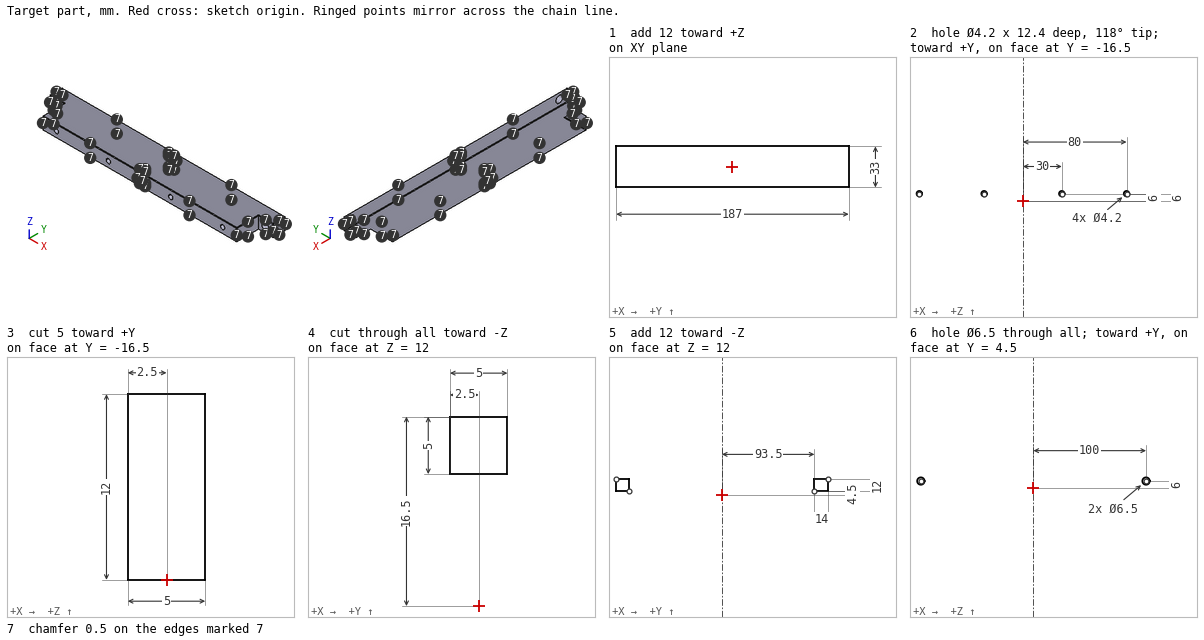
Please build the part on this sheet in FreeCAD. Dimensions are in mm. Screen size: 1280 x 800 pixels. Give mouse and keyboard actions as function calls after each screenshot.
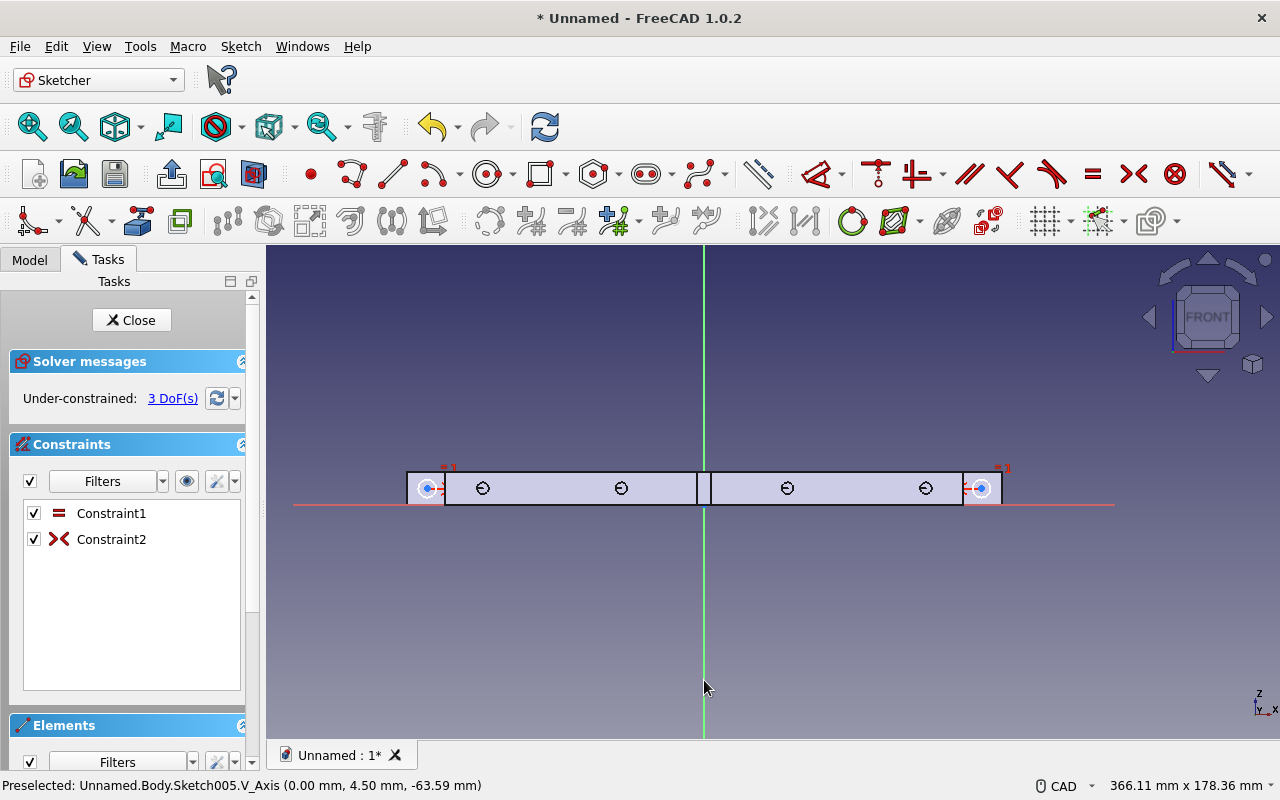
click(816, 174)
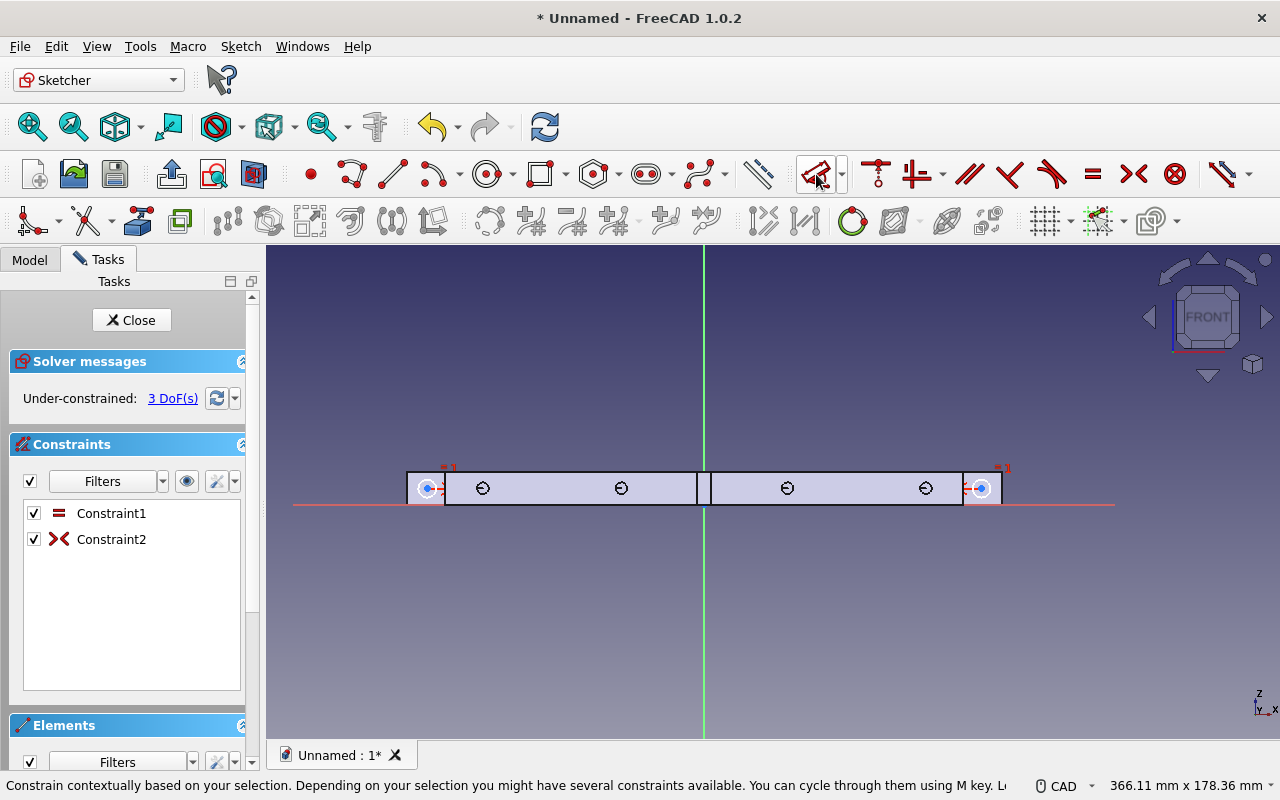
scroll(988, 495, up, 4)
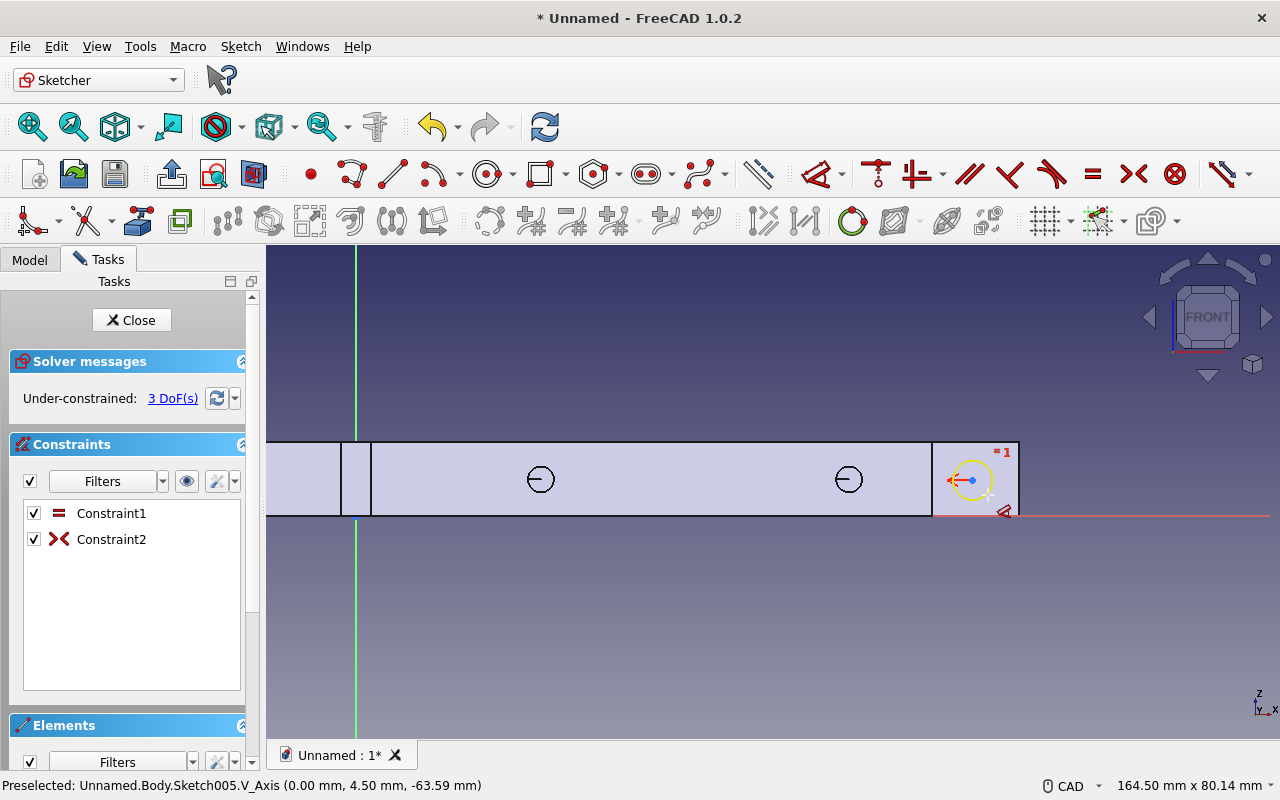
click(987, 494)
click(988, 530)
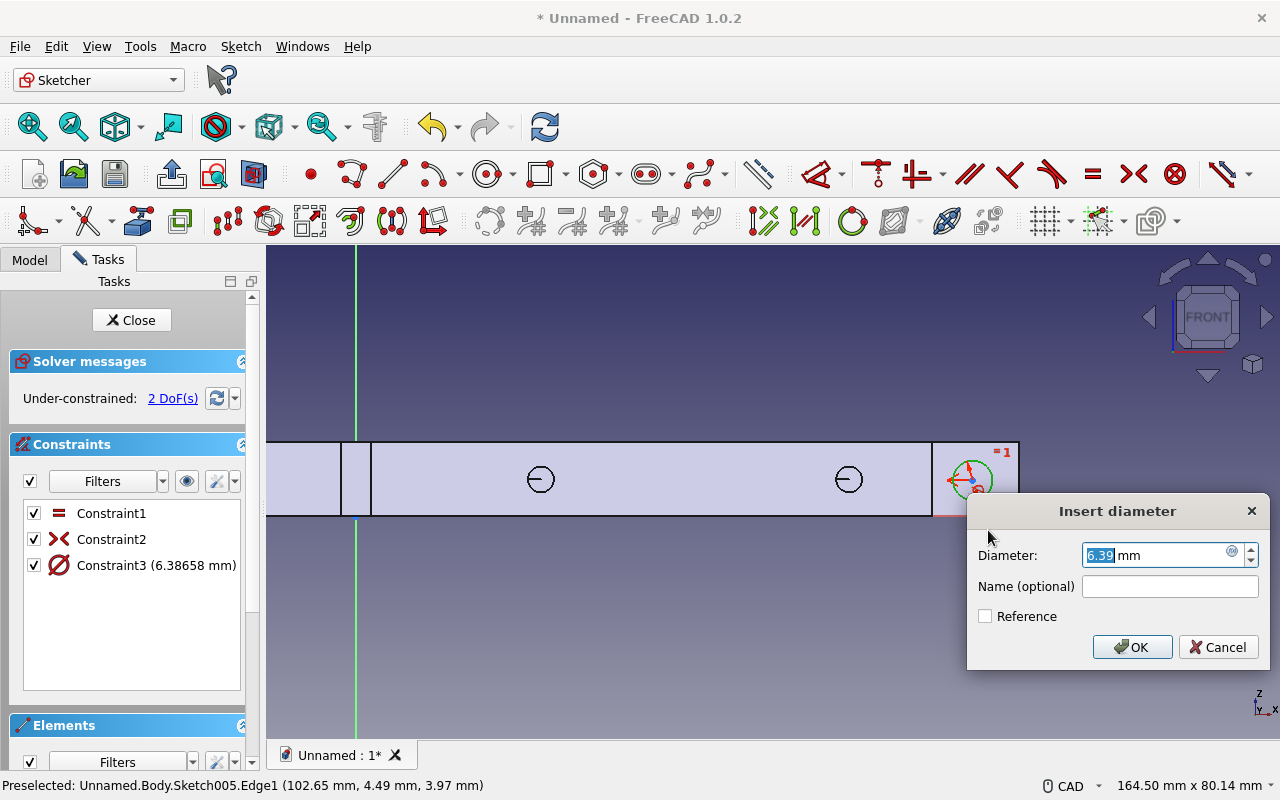
text(6.5)
key(Return)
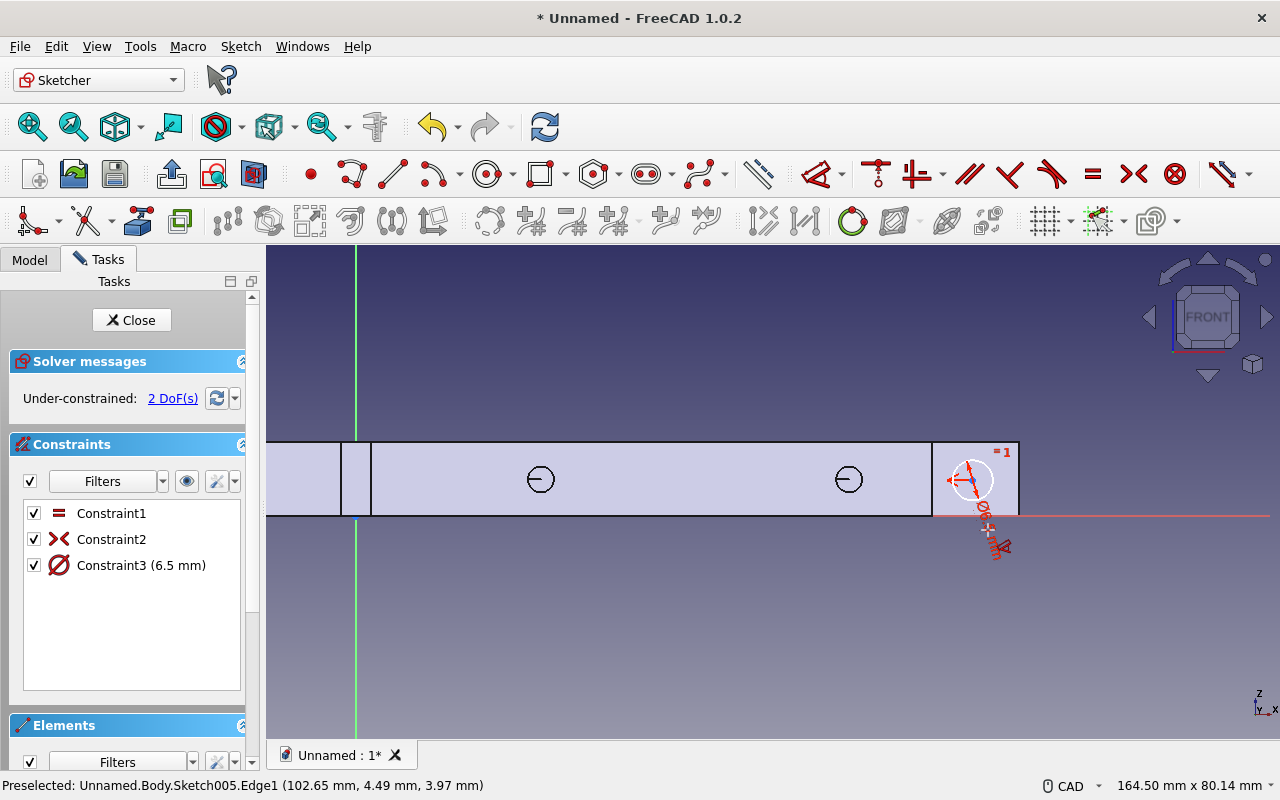
click(973, 480)
click(1007, 498)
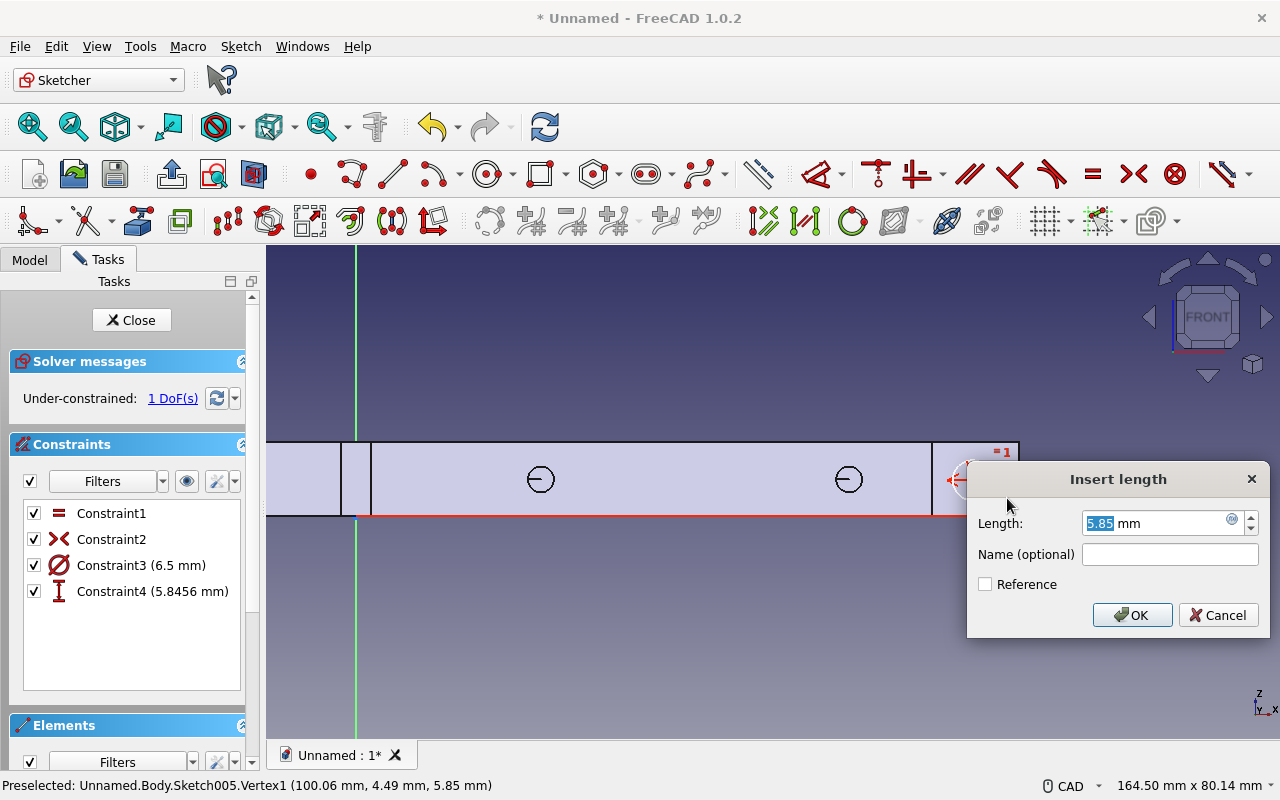
text(6)
key(Return)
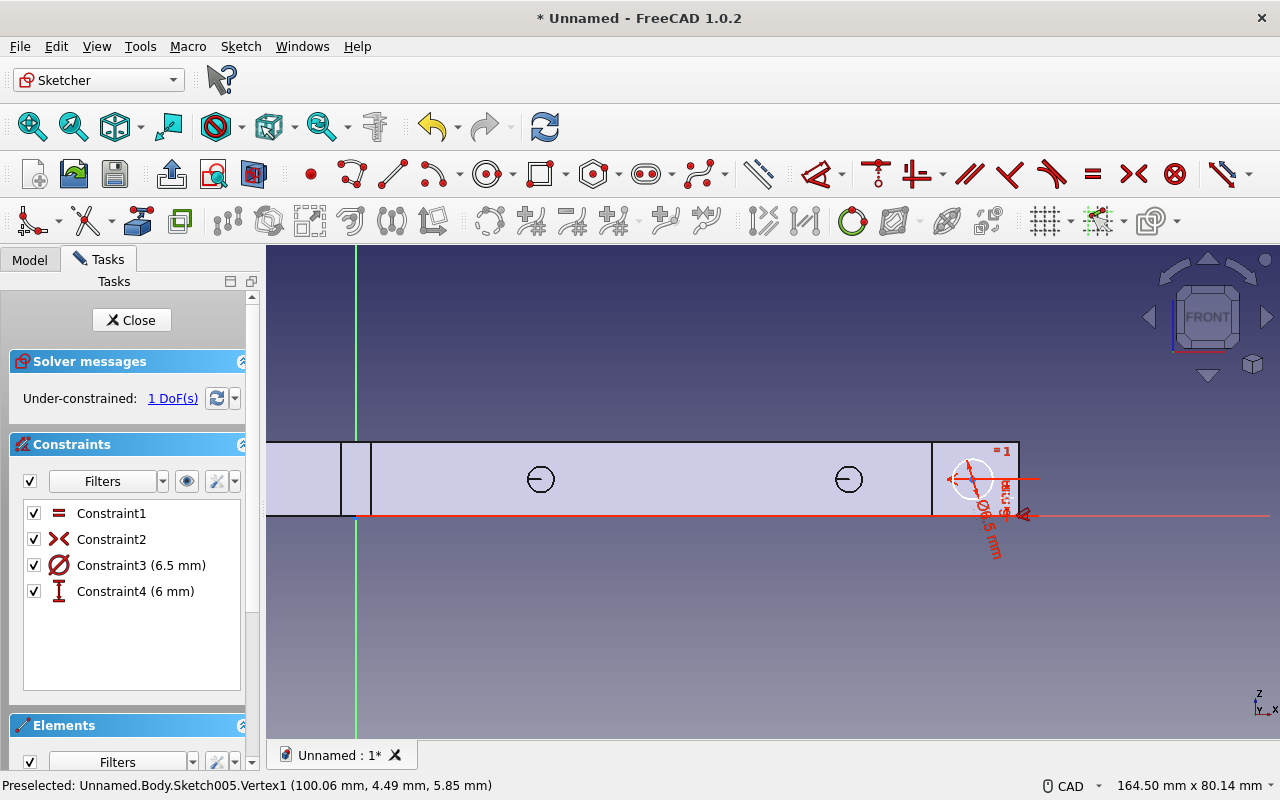
click(973, 479)
click(664, 550)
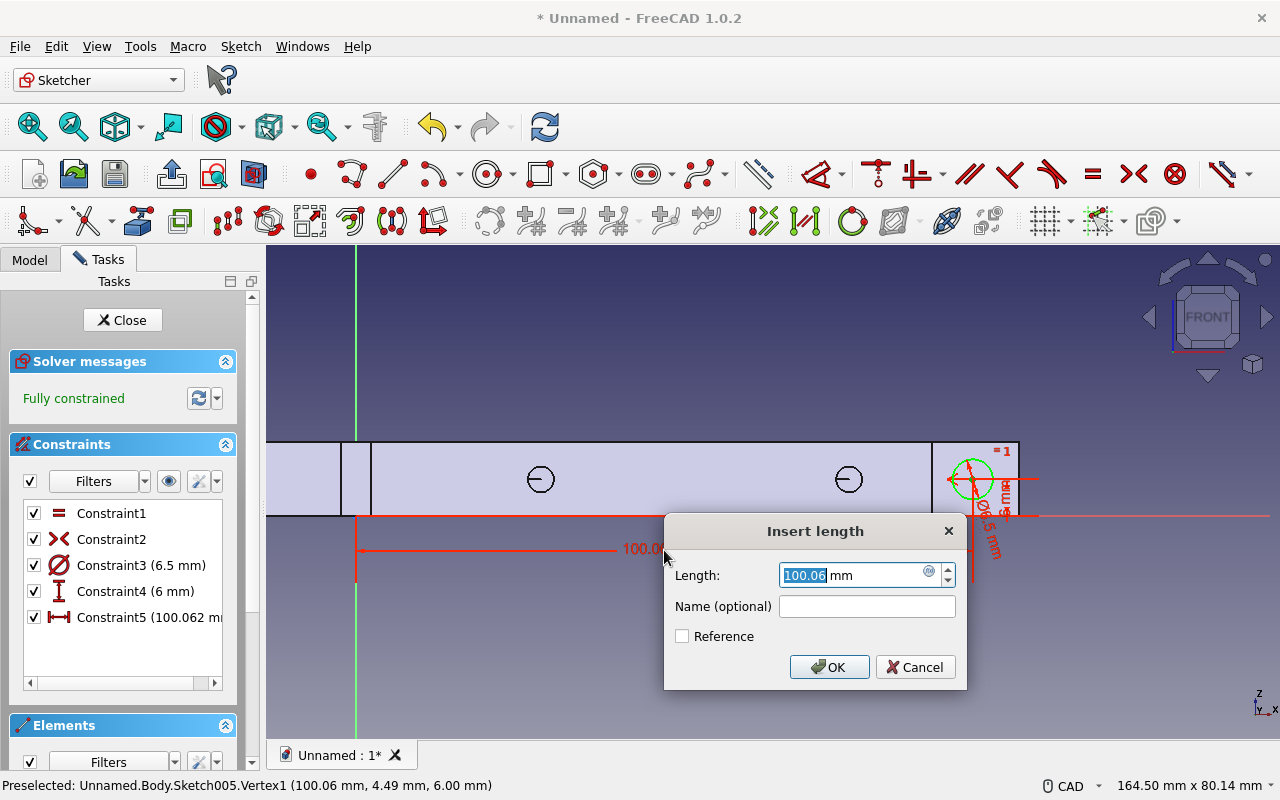
text(100)
key(Return)
key(Escape)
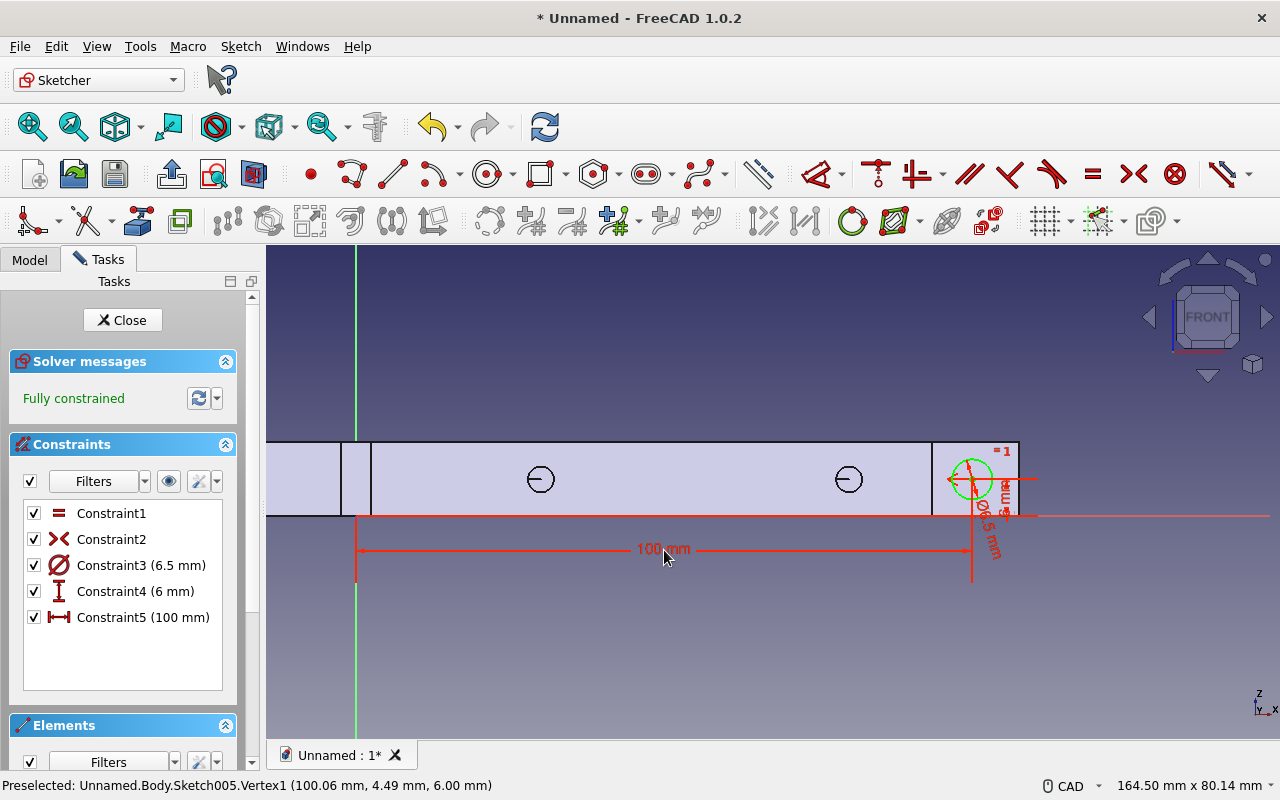
click(123, 320)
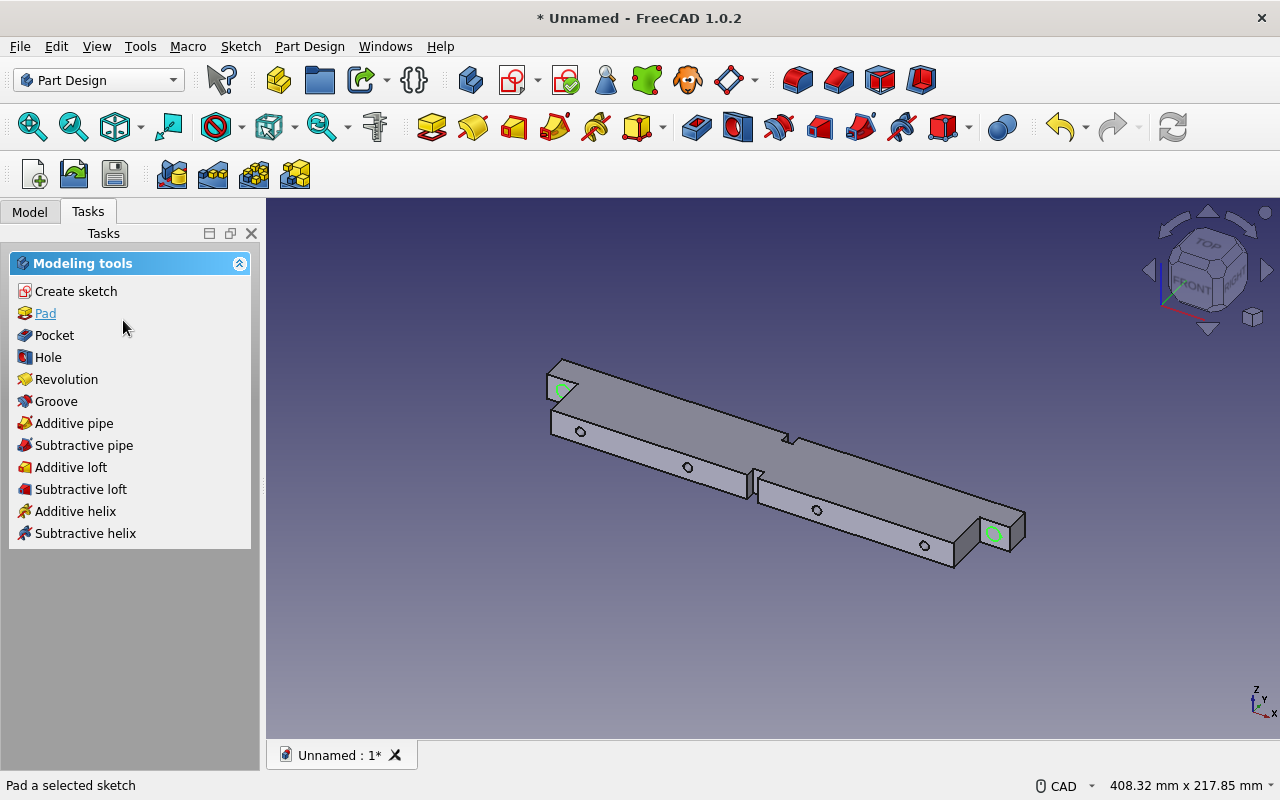
click(738, 128)